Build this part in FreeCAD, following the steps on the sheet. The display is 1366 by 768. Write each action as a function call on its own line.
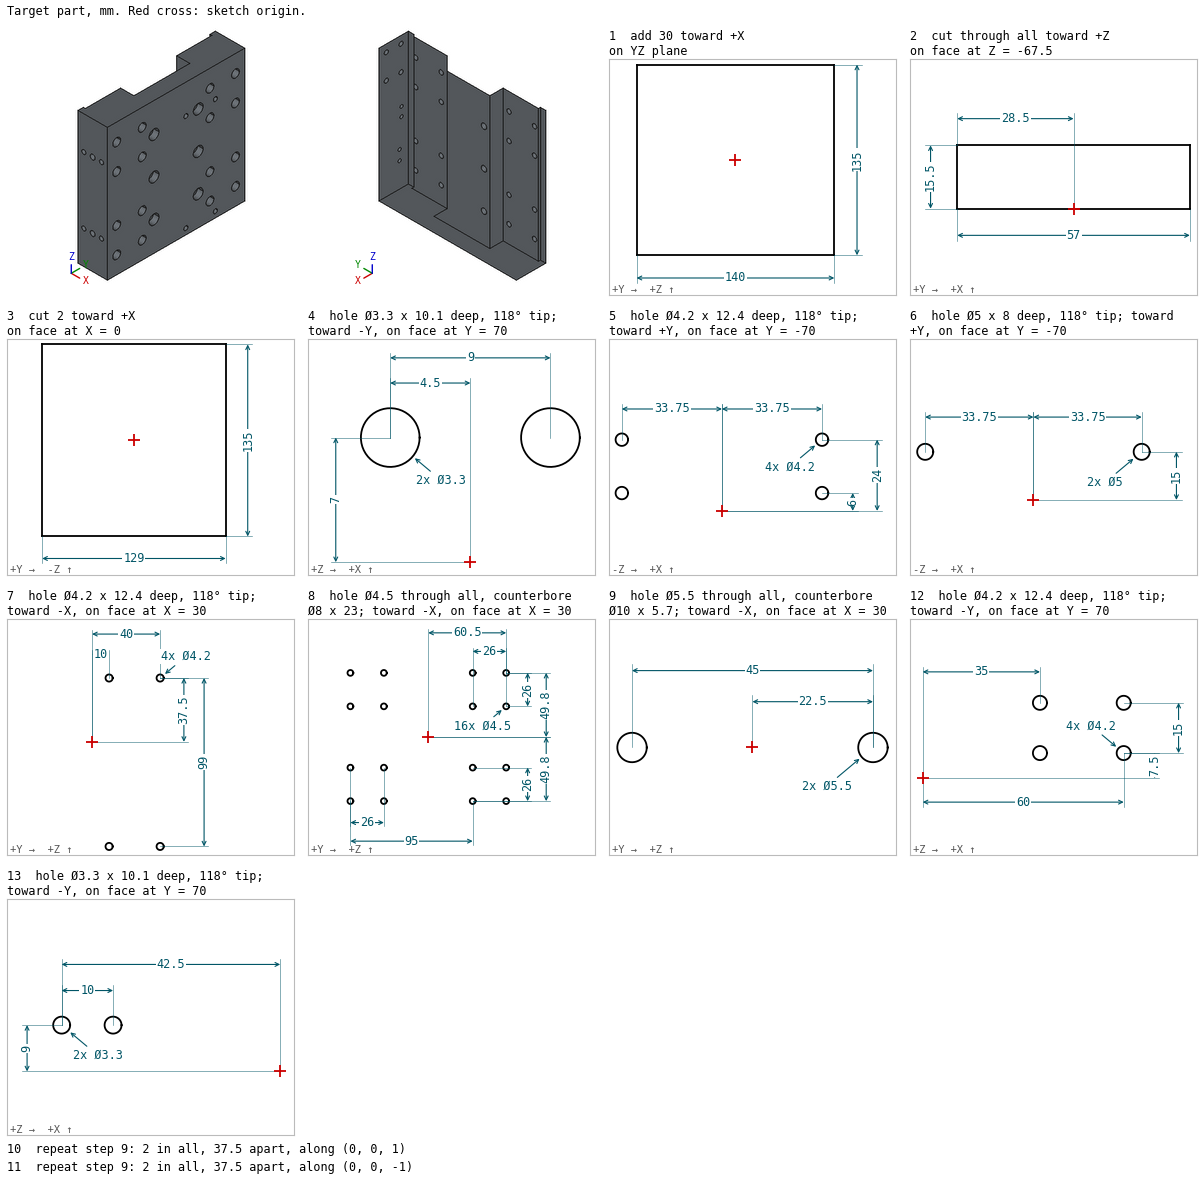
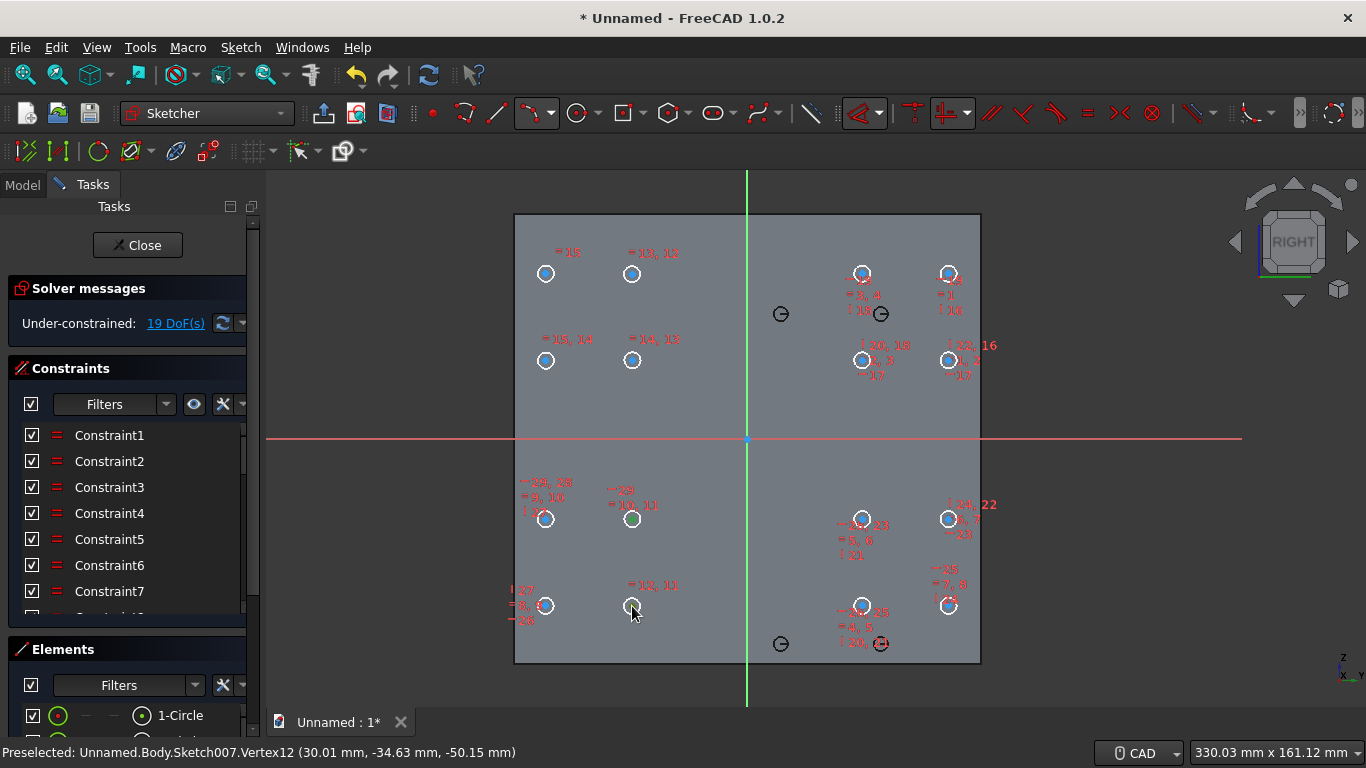
key(v)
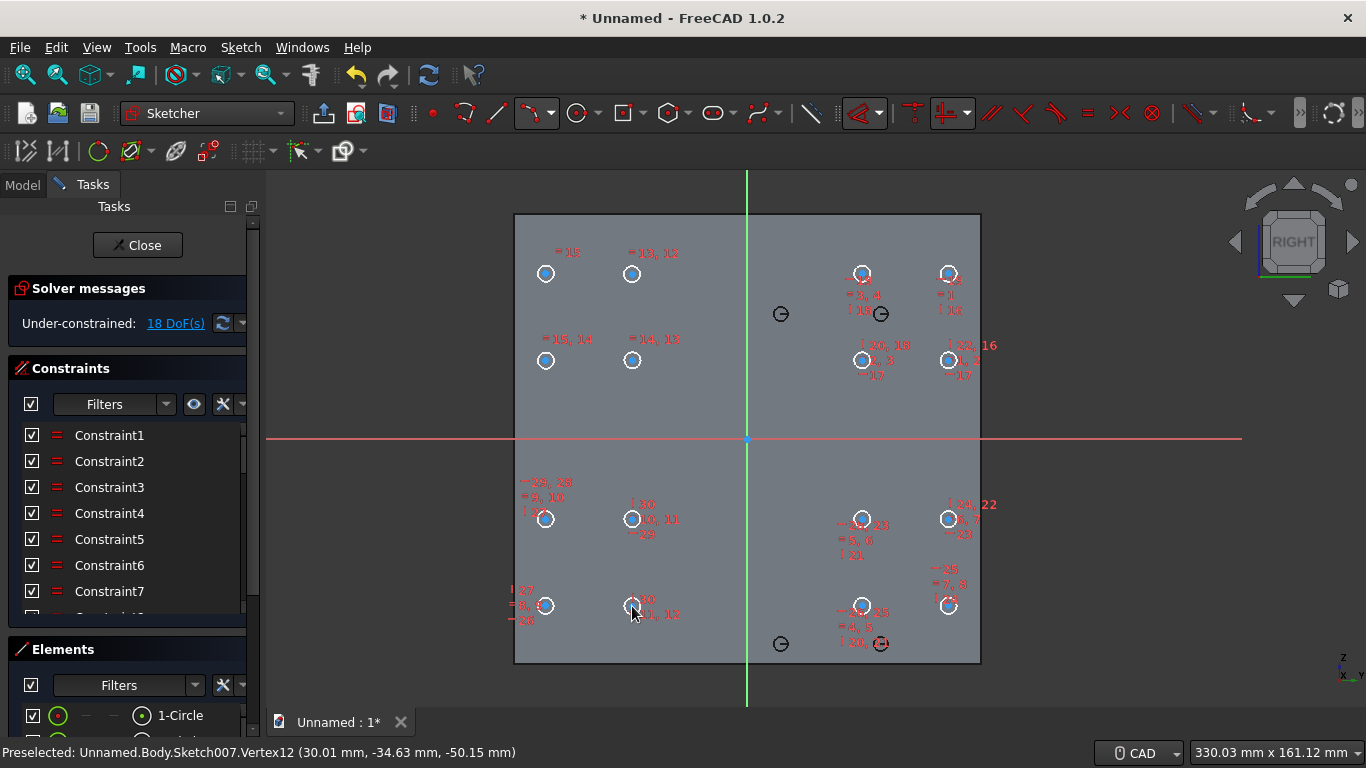
click(546, 606)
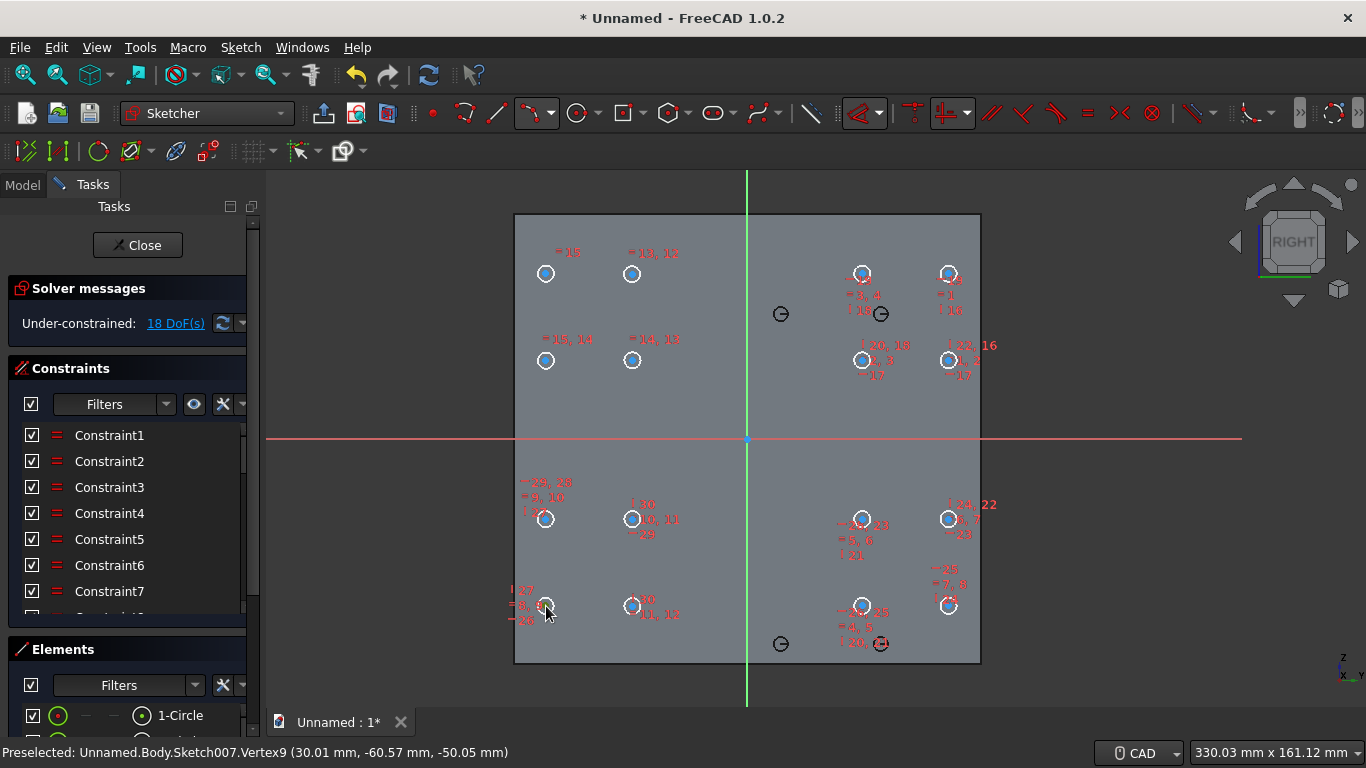
scroll(632, 606, up, 4)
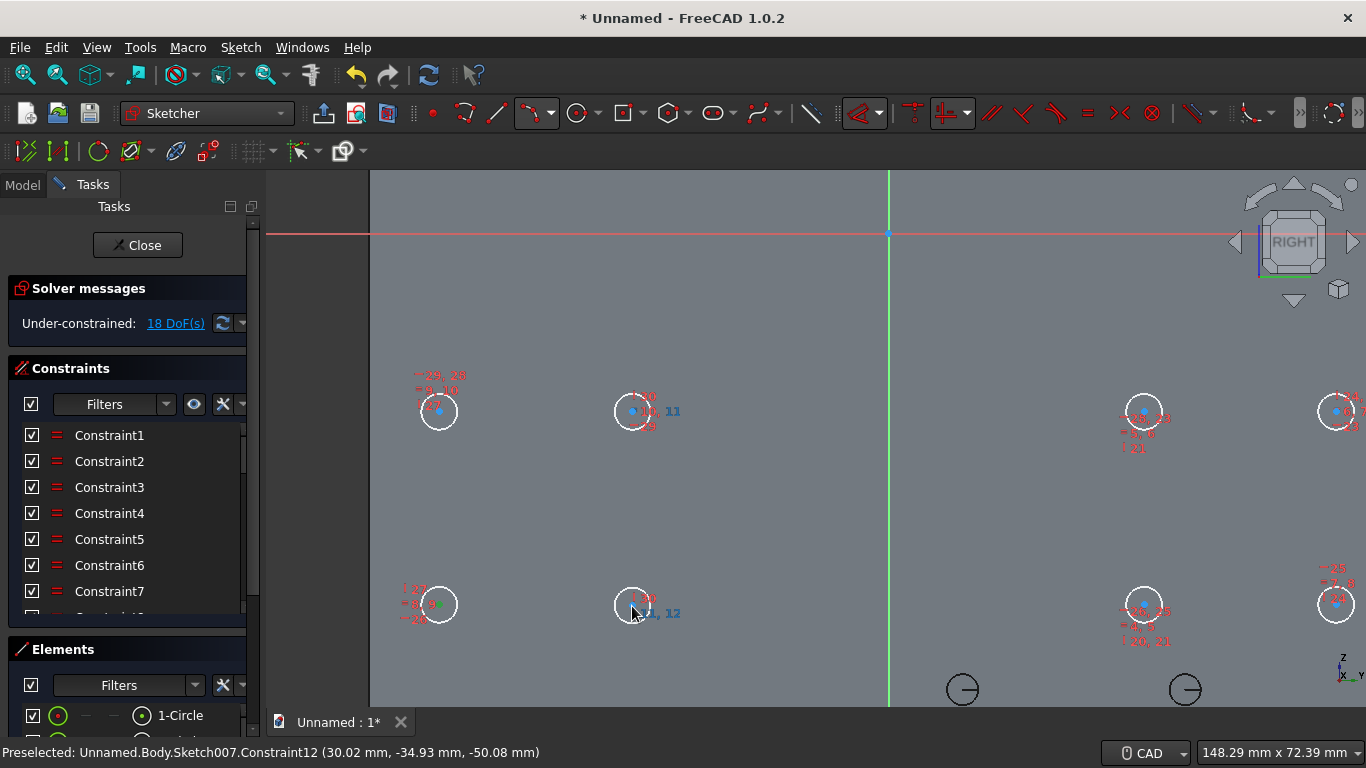
scroll(633, 606, up, 4)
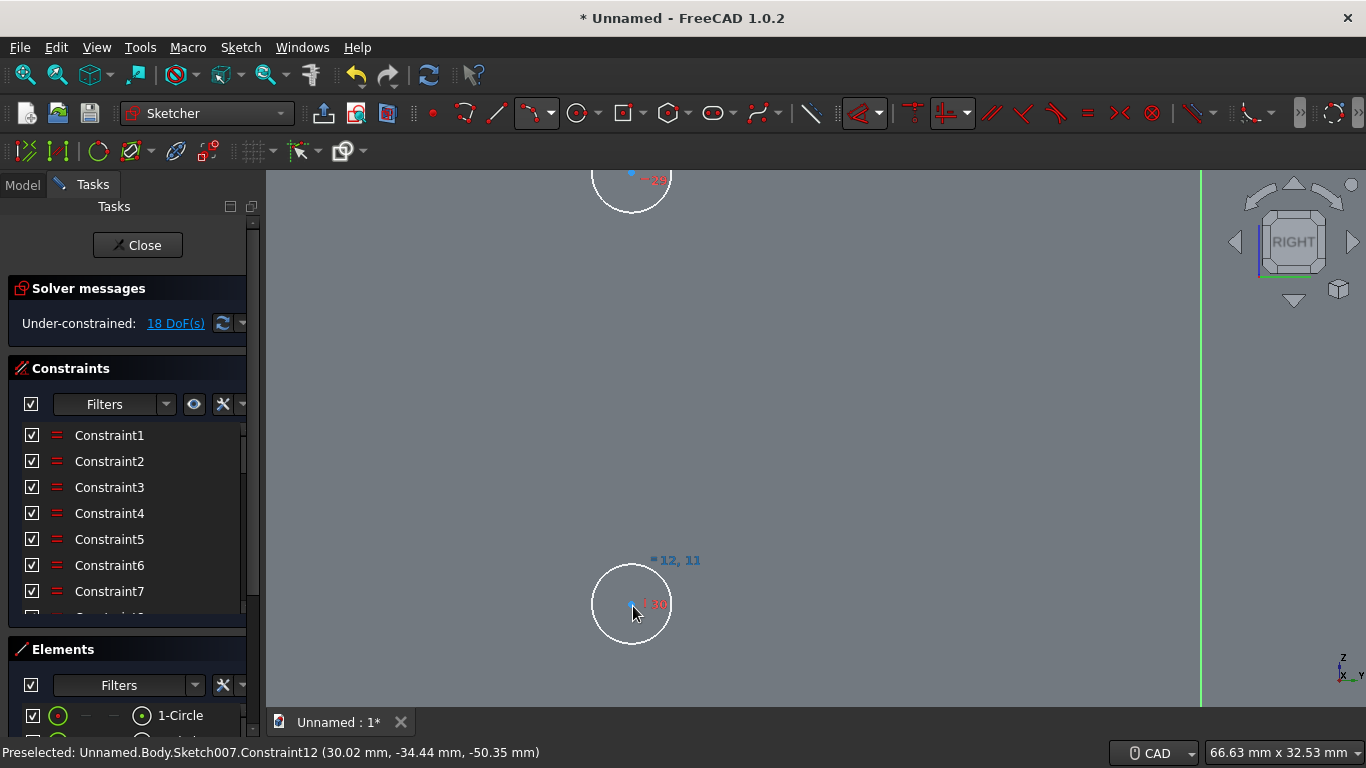
click(632, 604)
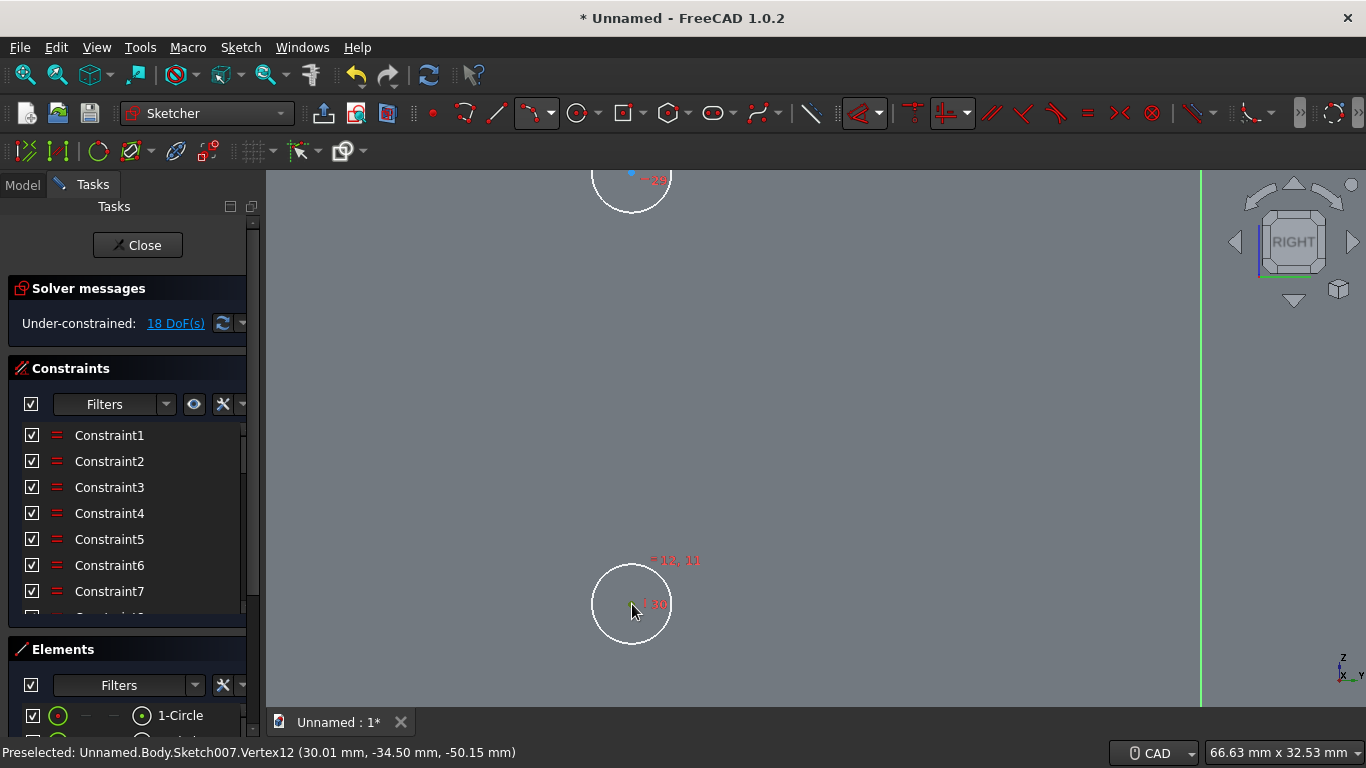
key(h)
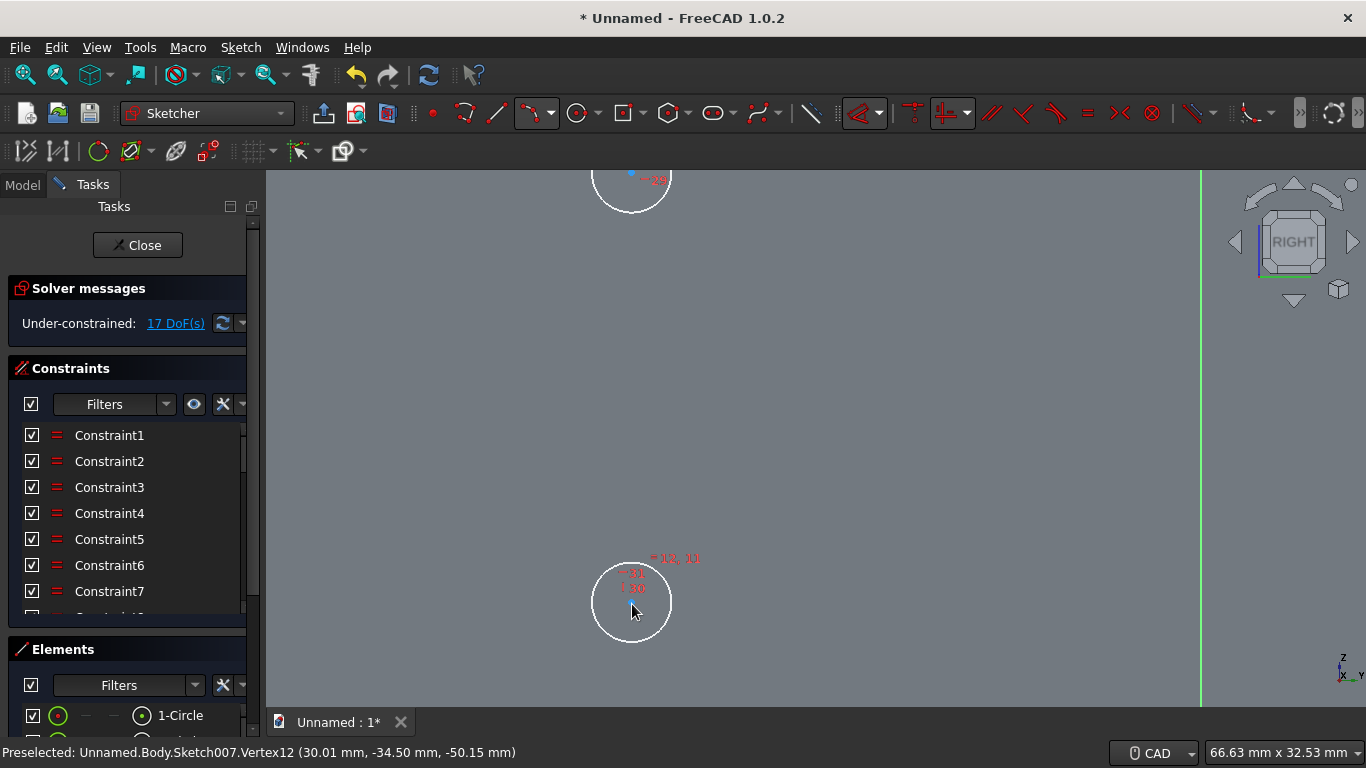
scroll(633, 606, down, 8)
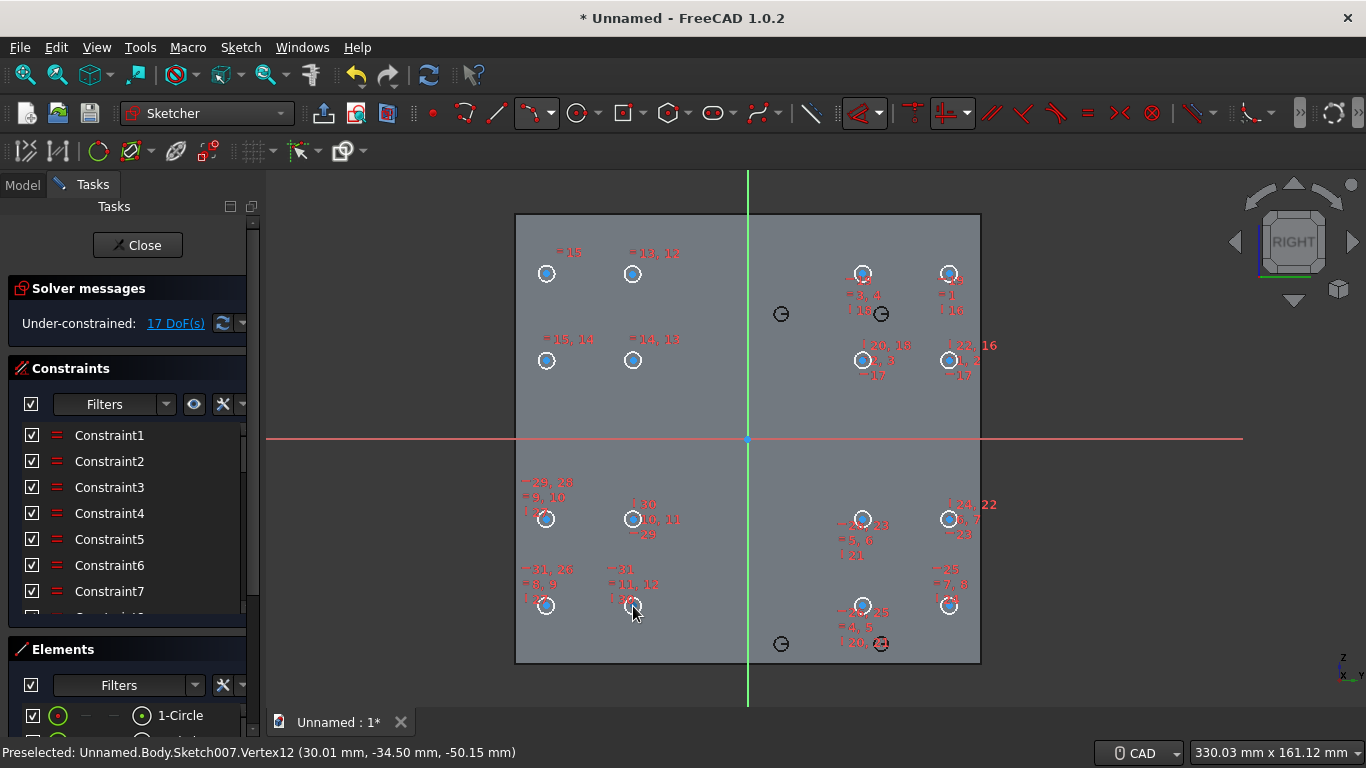
click(633, 519)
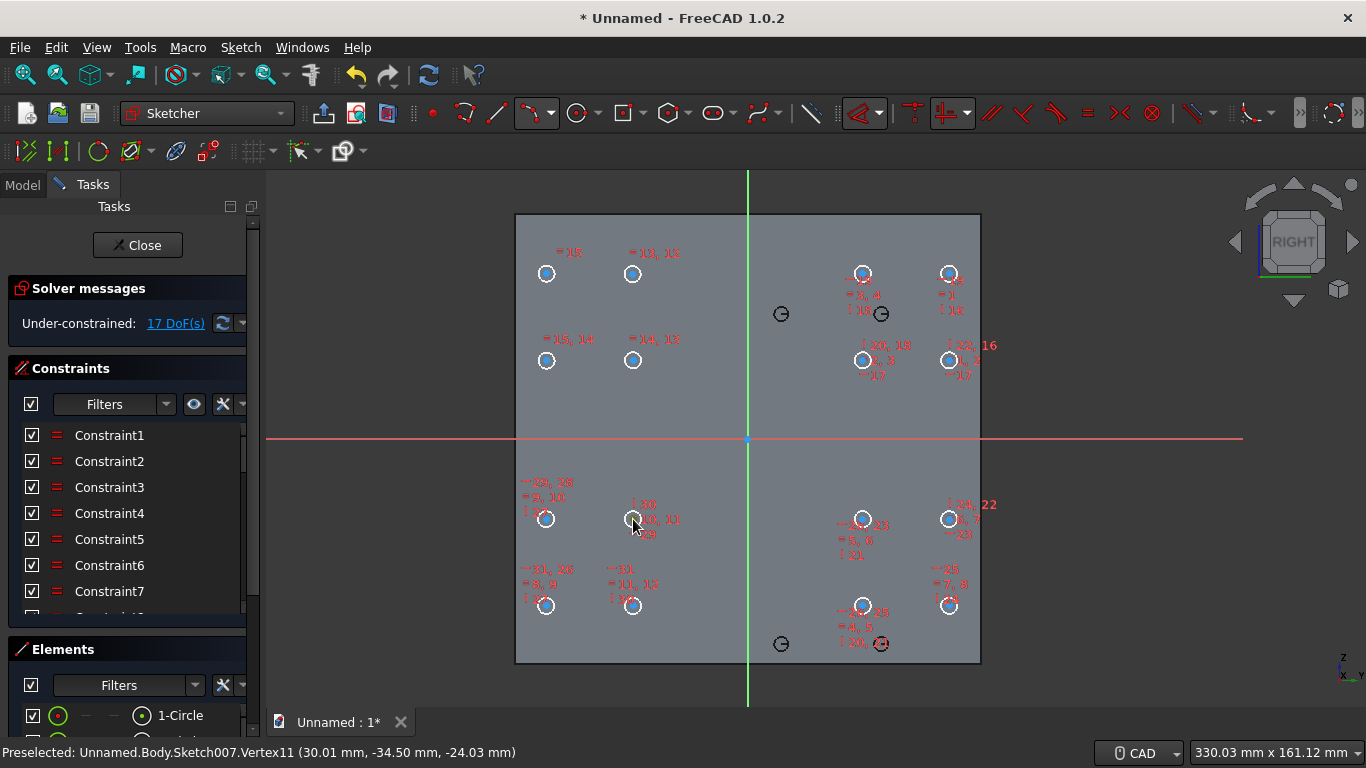
click(633, 274)